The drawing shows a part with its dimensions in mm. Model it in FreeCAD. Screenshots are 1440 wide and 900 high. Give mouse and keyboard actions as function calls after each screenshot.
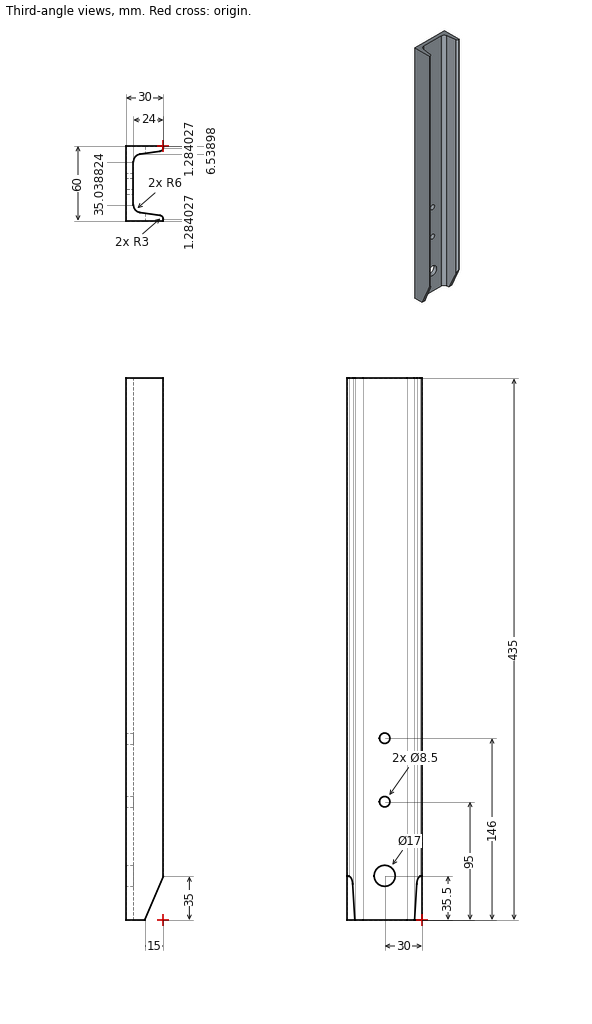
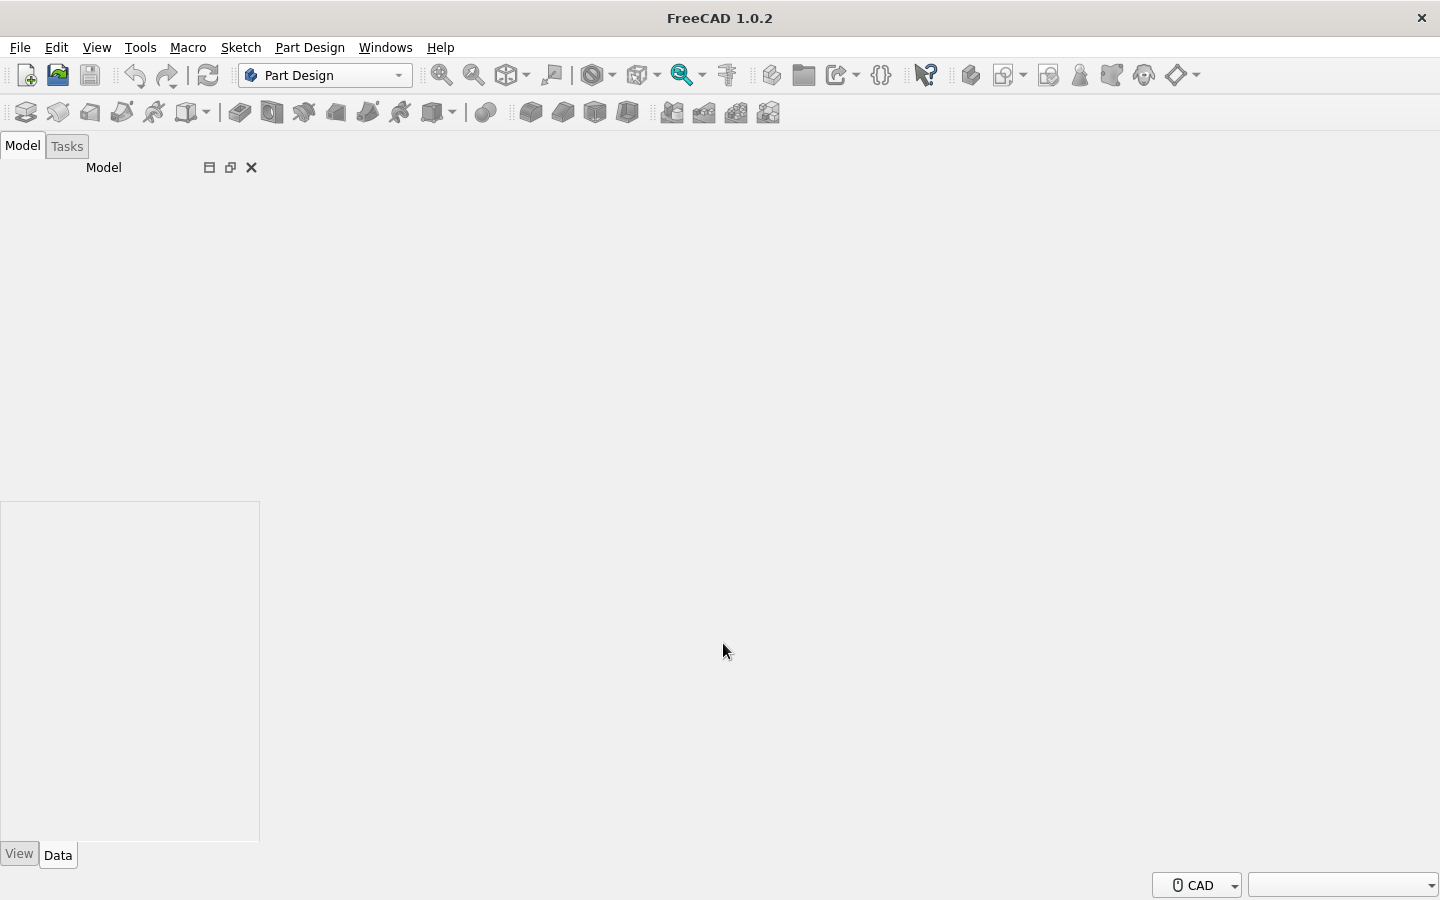
key(ctrl+n)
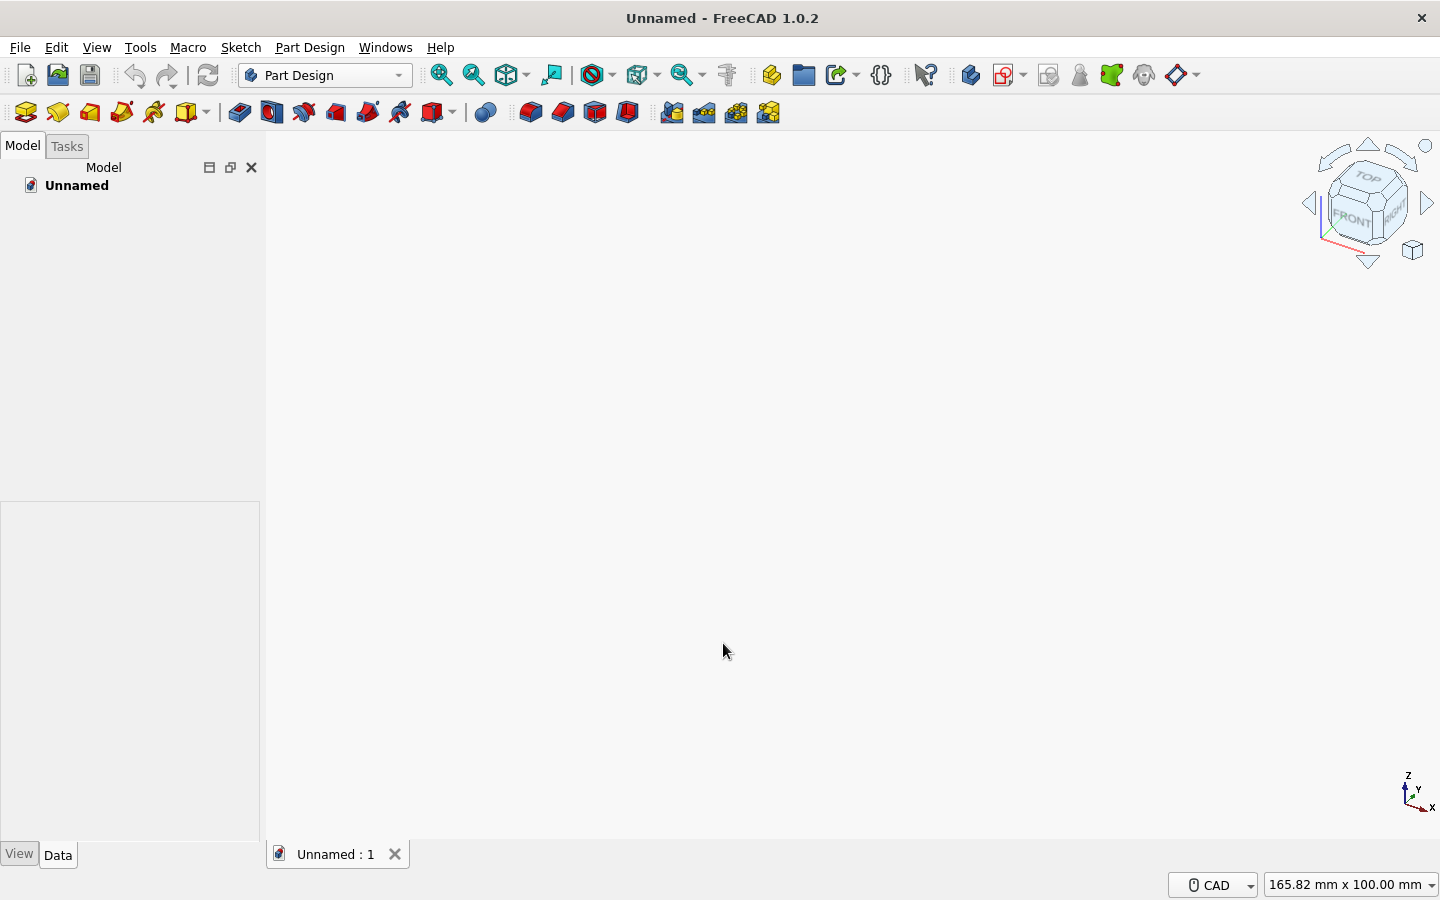
click(1004, 76)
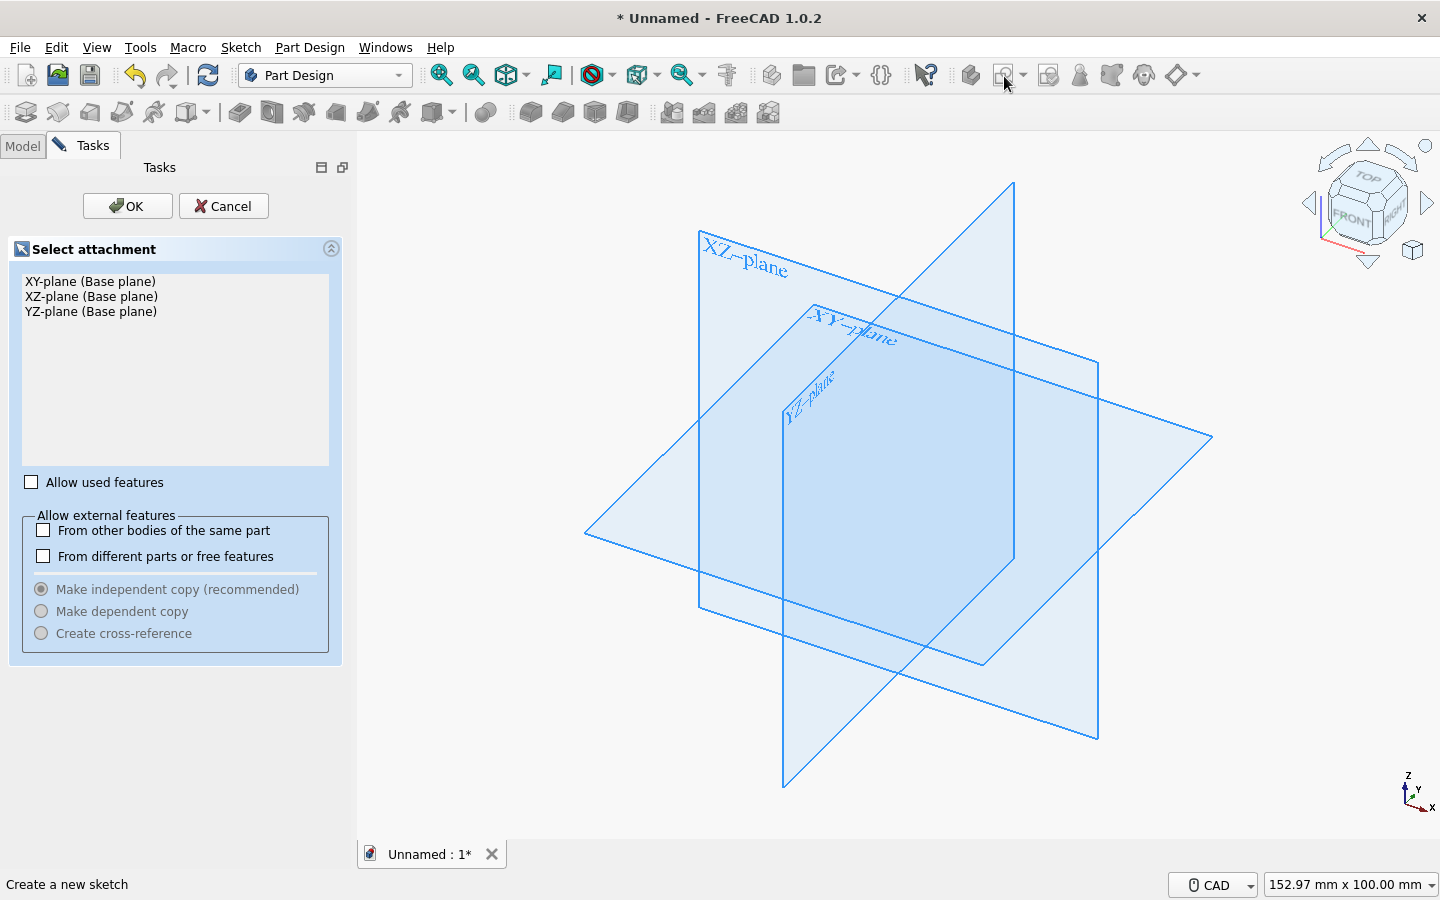
click(82, 282)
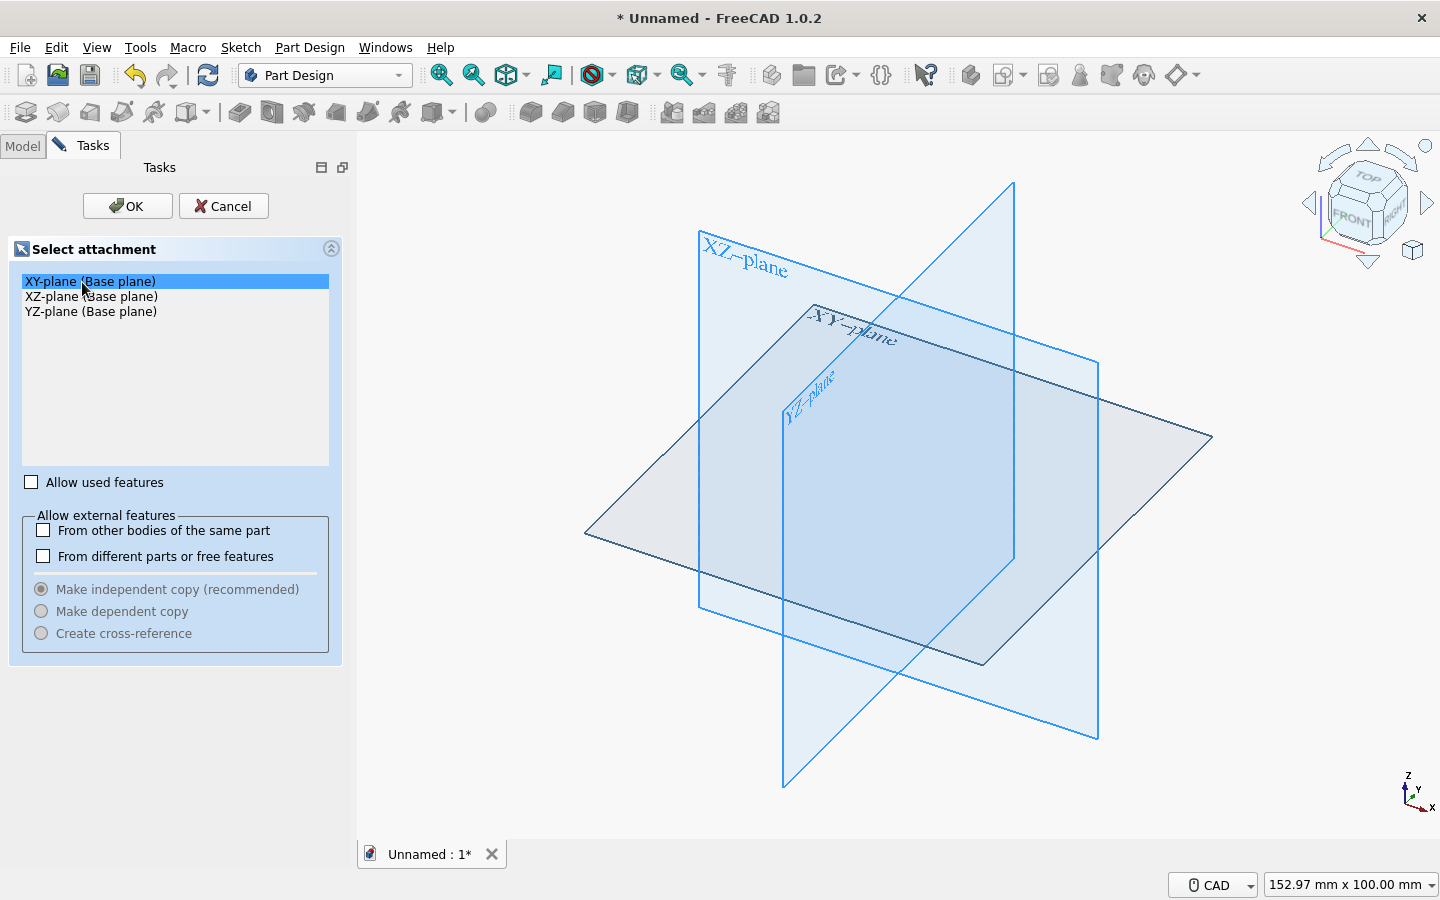
click(128, 206)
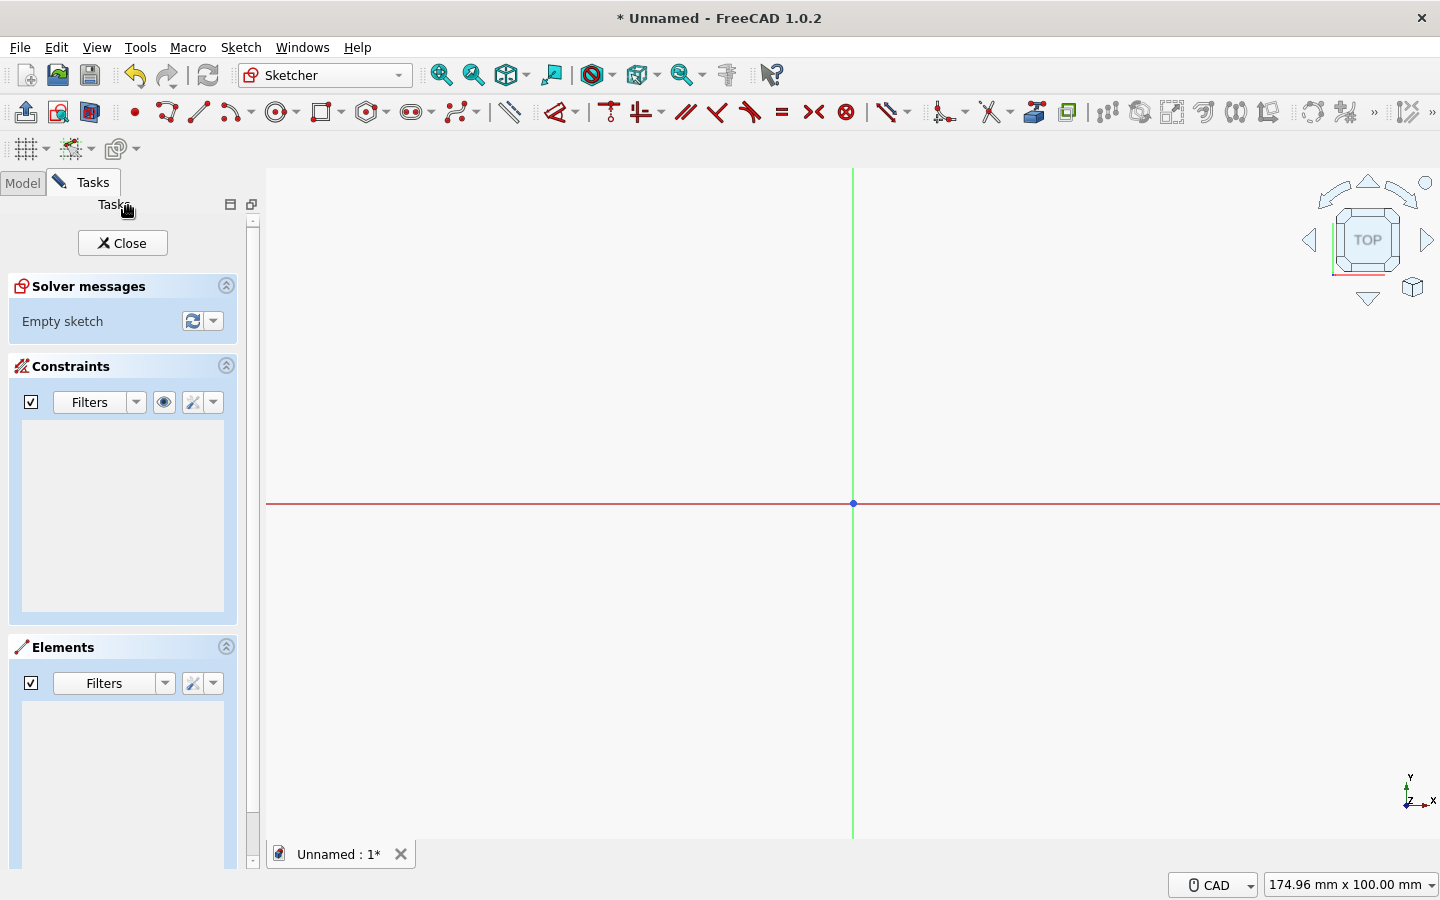
scroll(930, 196, down, 1)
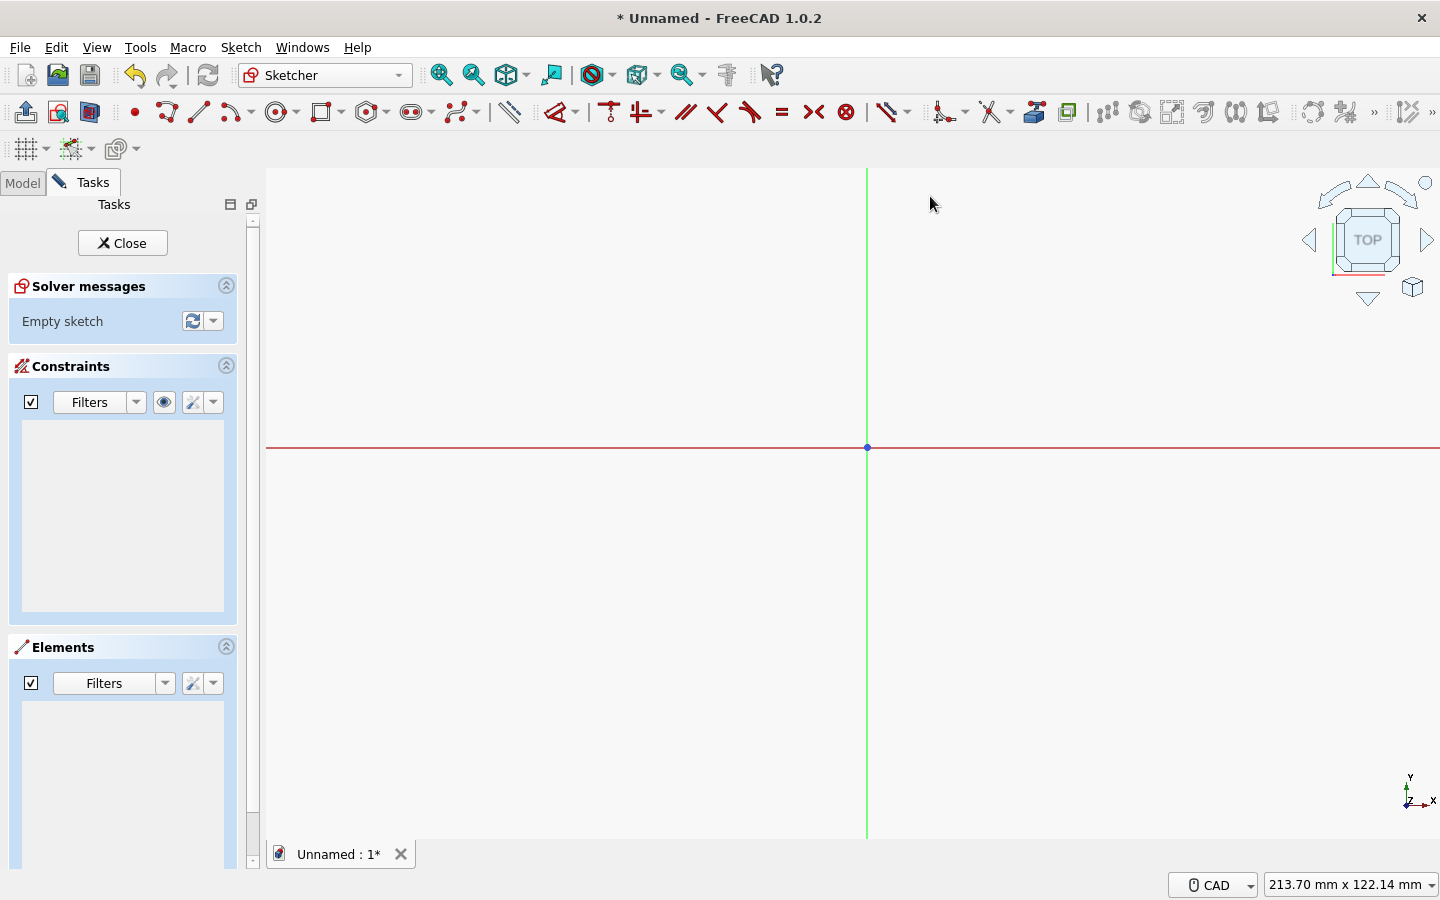
click(200, 112)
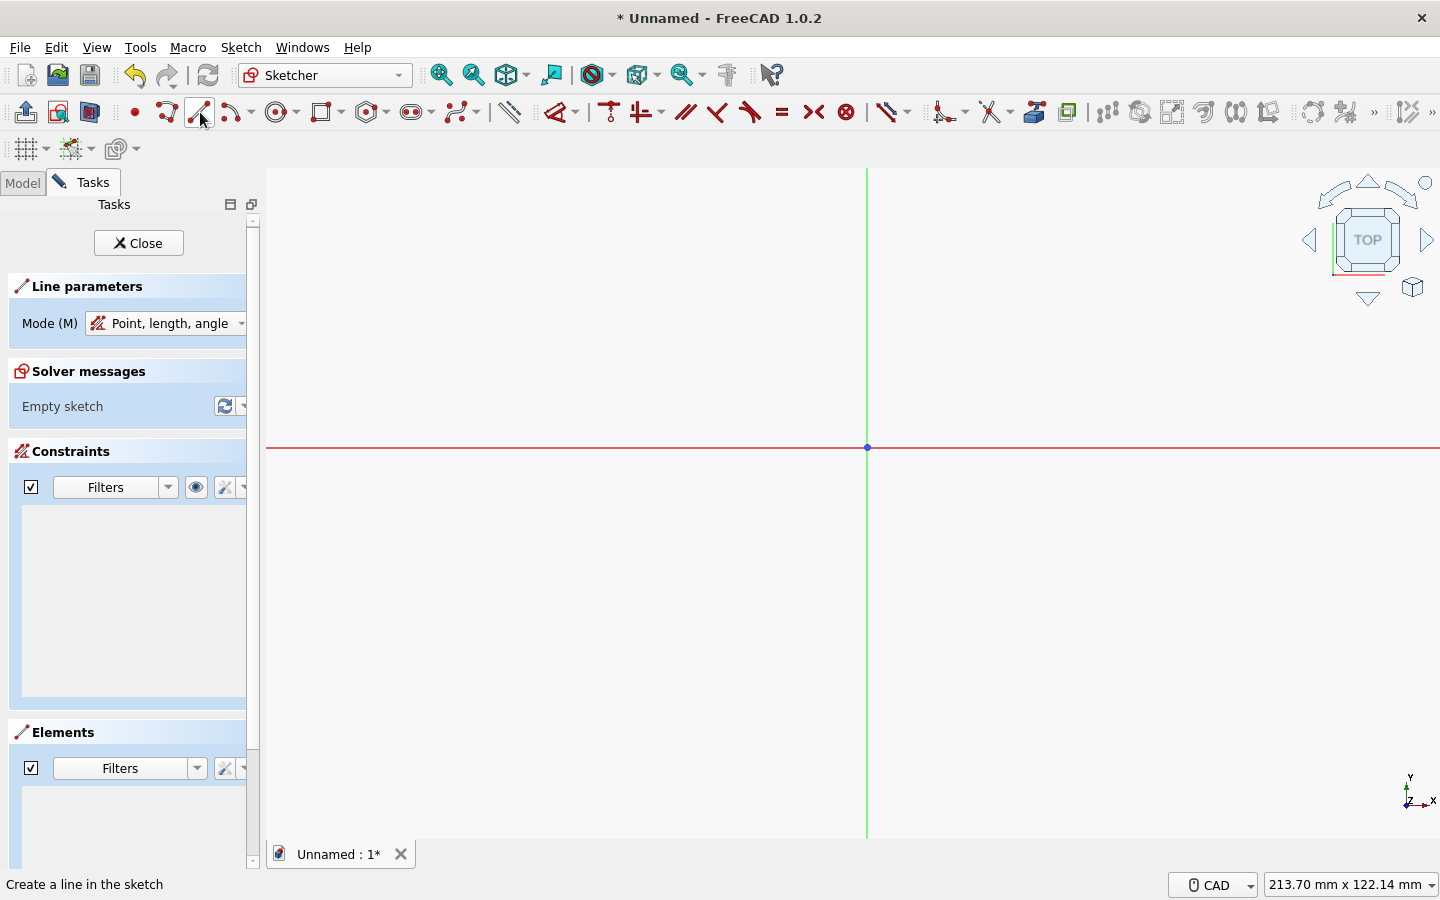
click(853, 754)
click(764, 741)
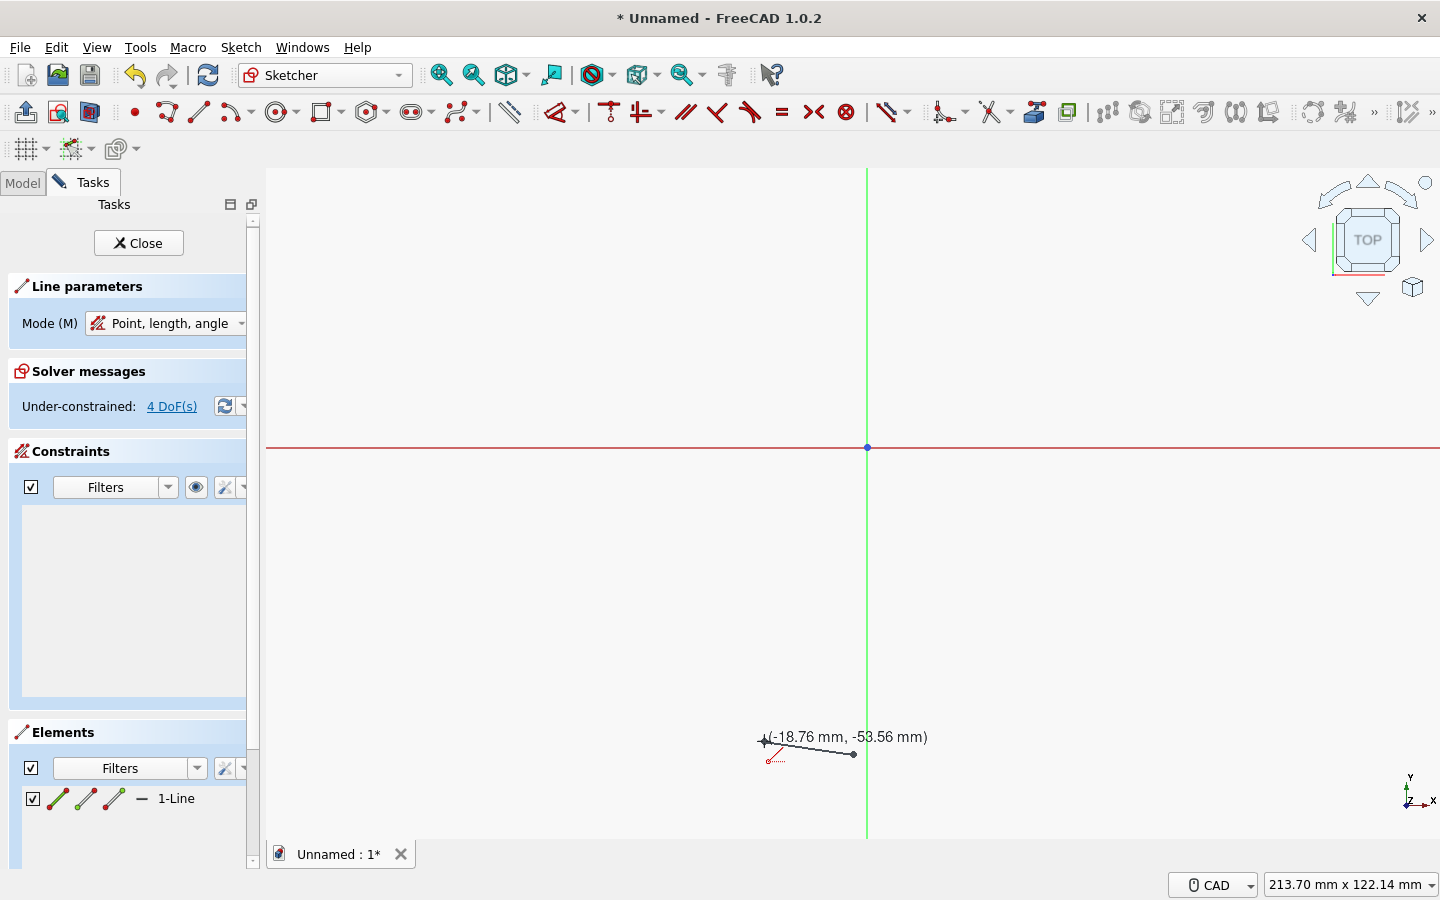
click(735, 709)
click(735, 516)